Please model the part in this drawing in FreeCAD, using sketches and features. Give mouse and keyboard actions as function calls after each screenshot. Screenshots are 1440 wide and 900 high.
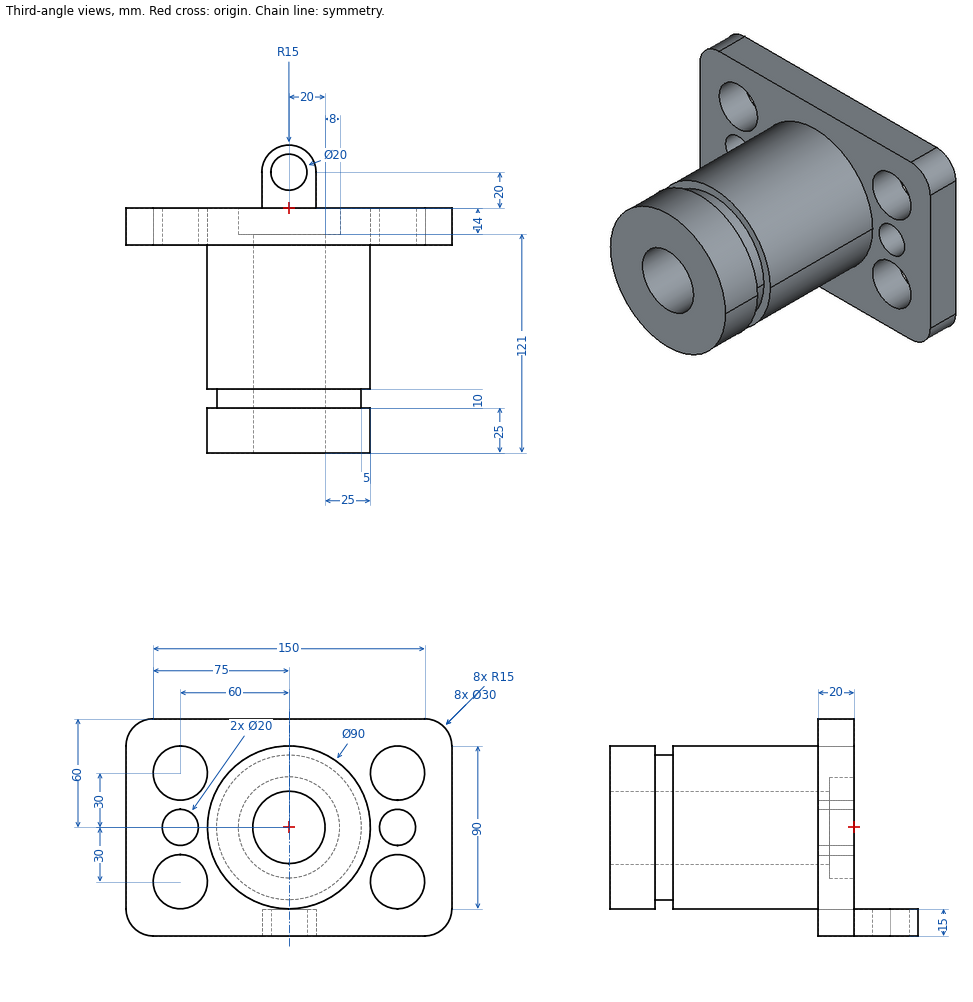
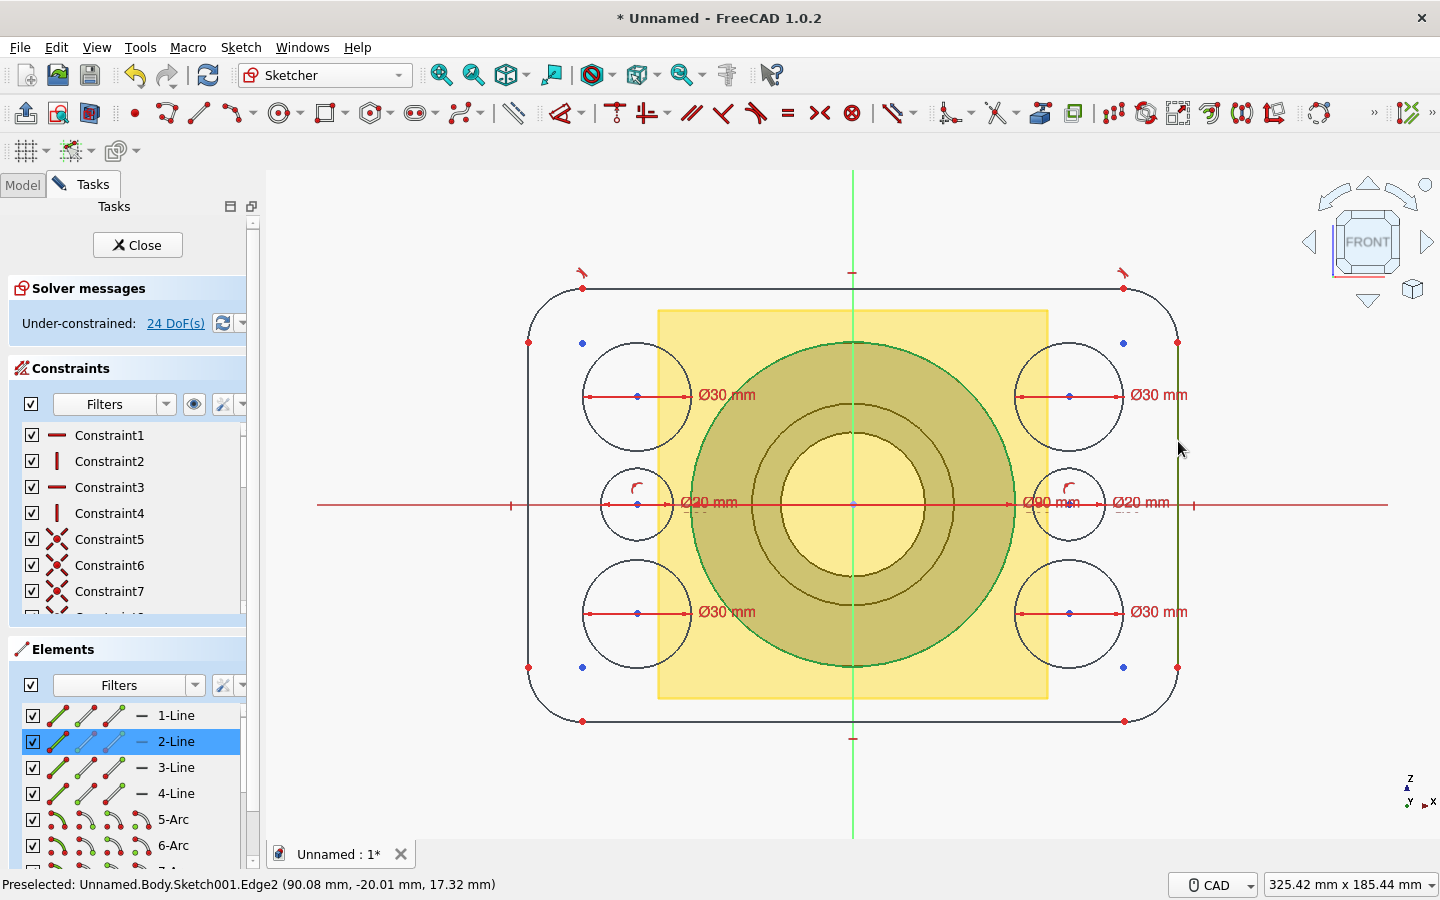
click(1172, 318)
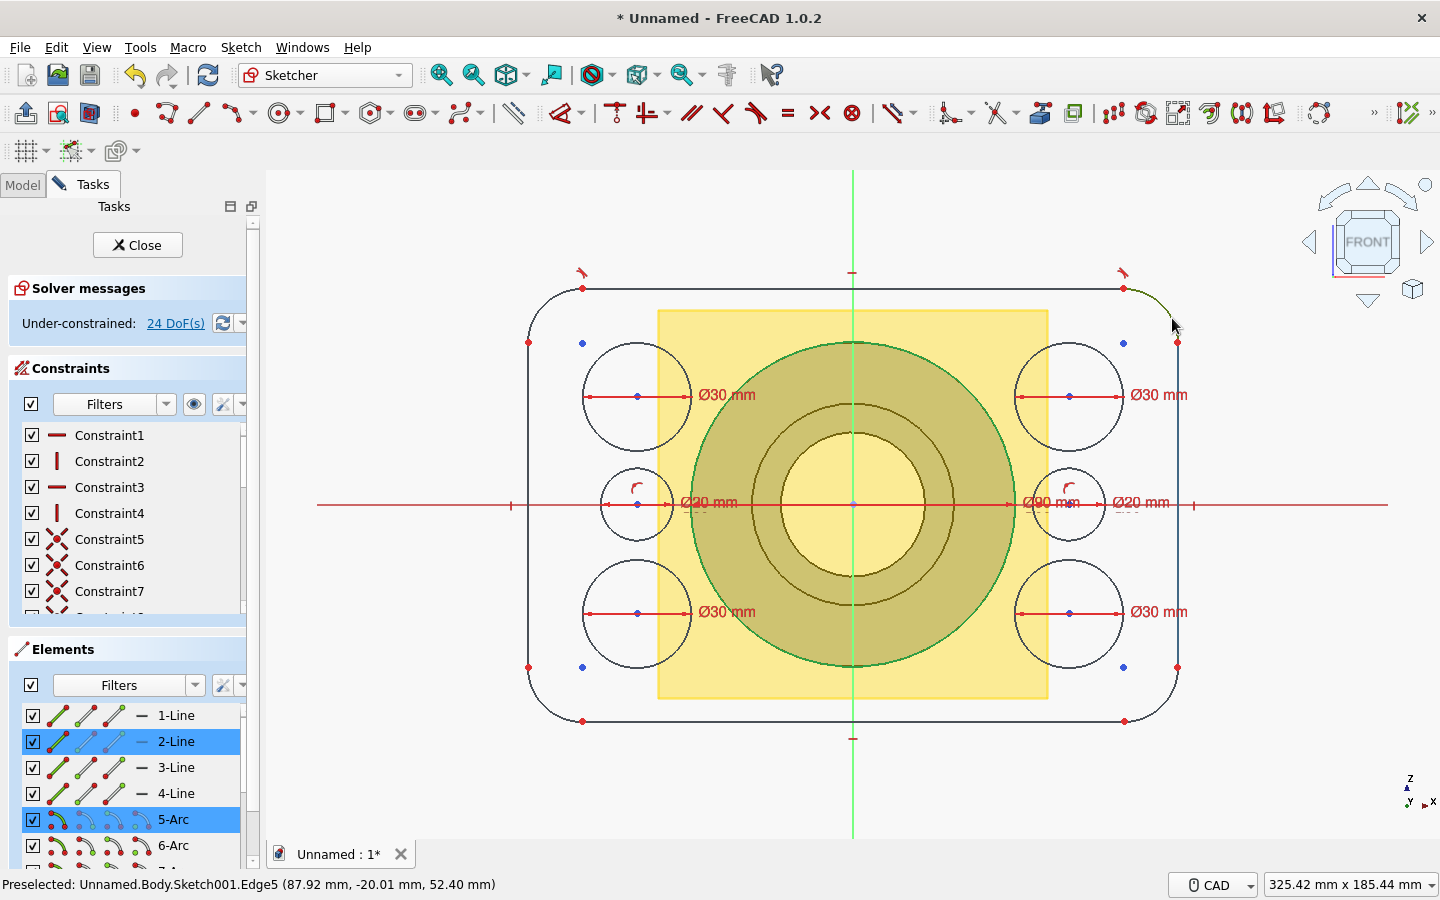
click(756, 114)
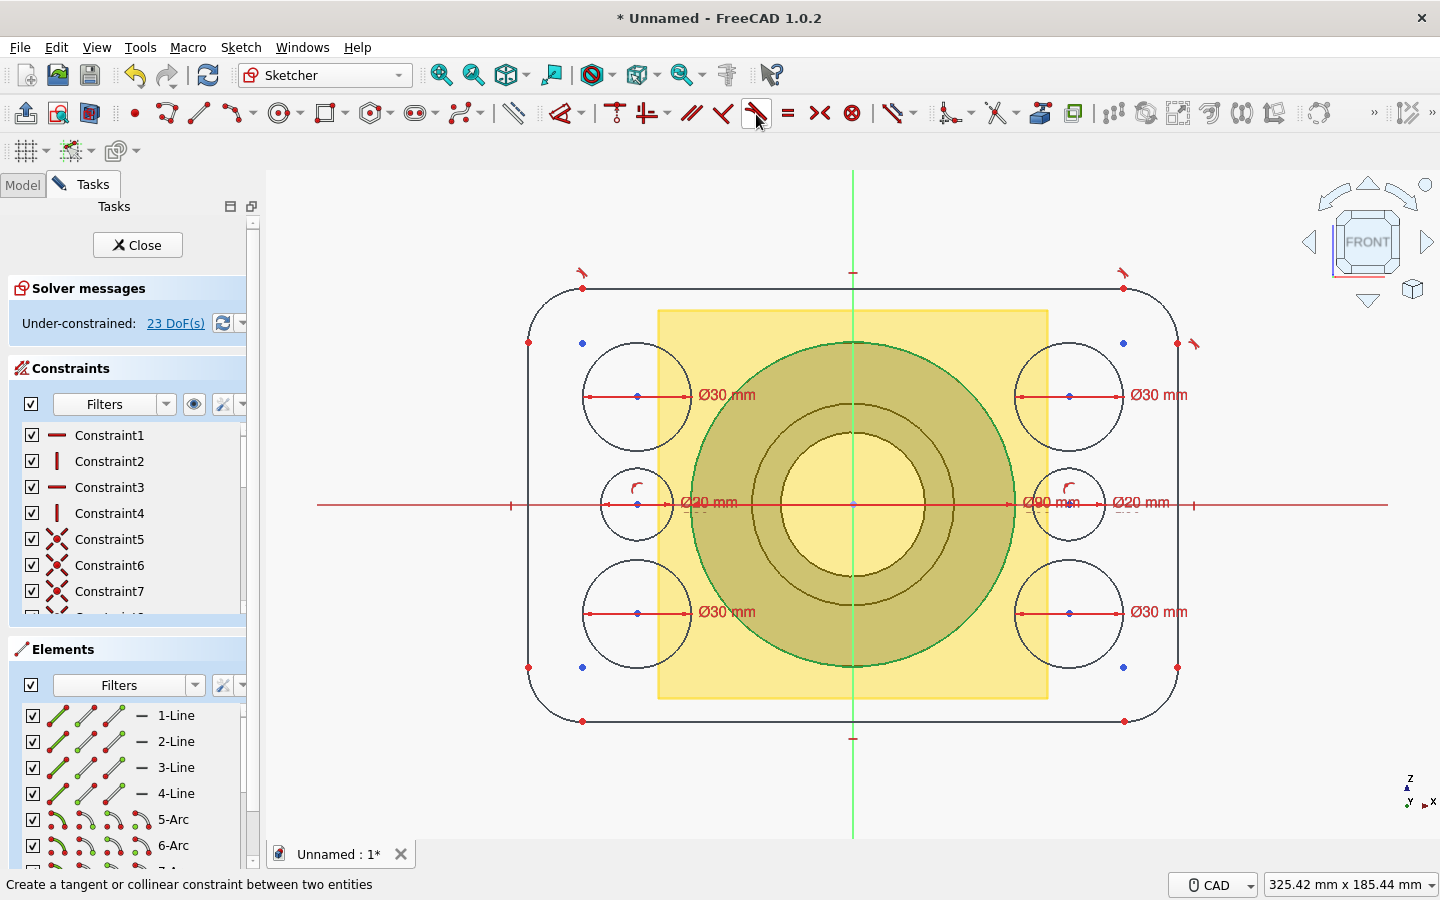
click(1178, 441)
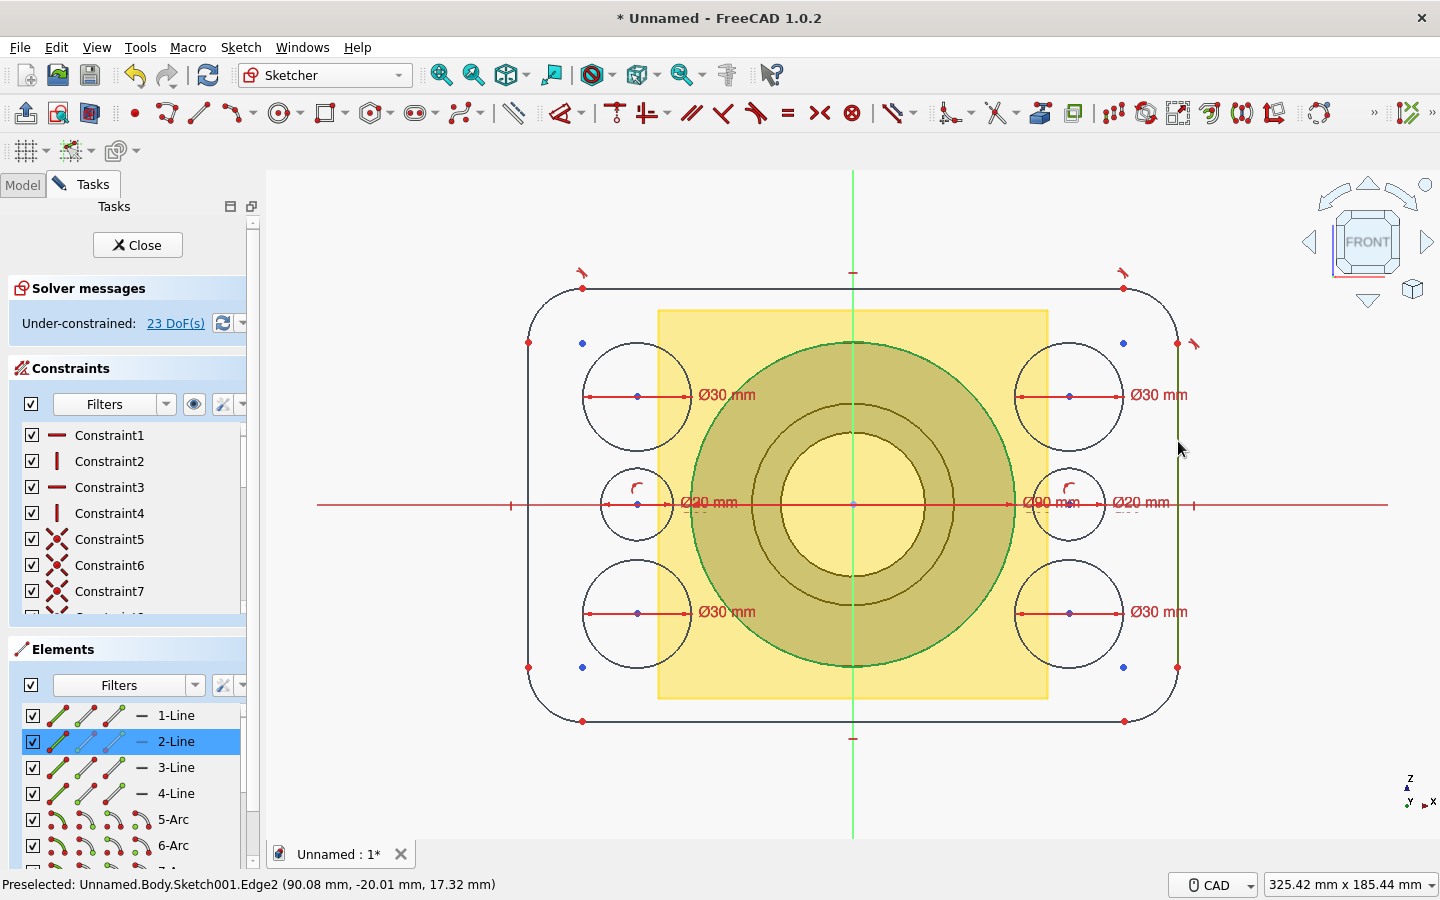
click(1148, 716)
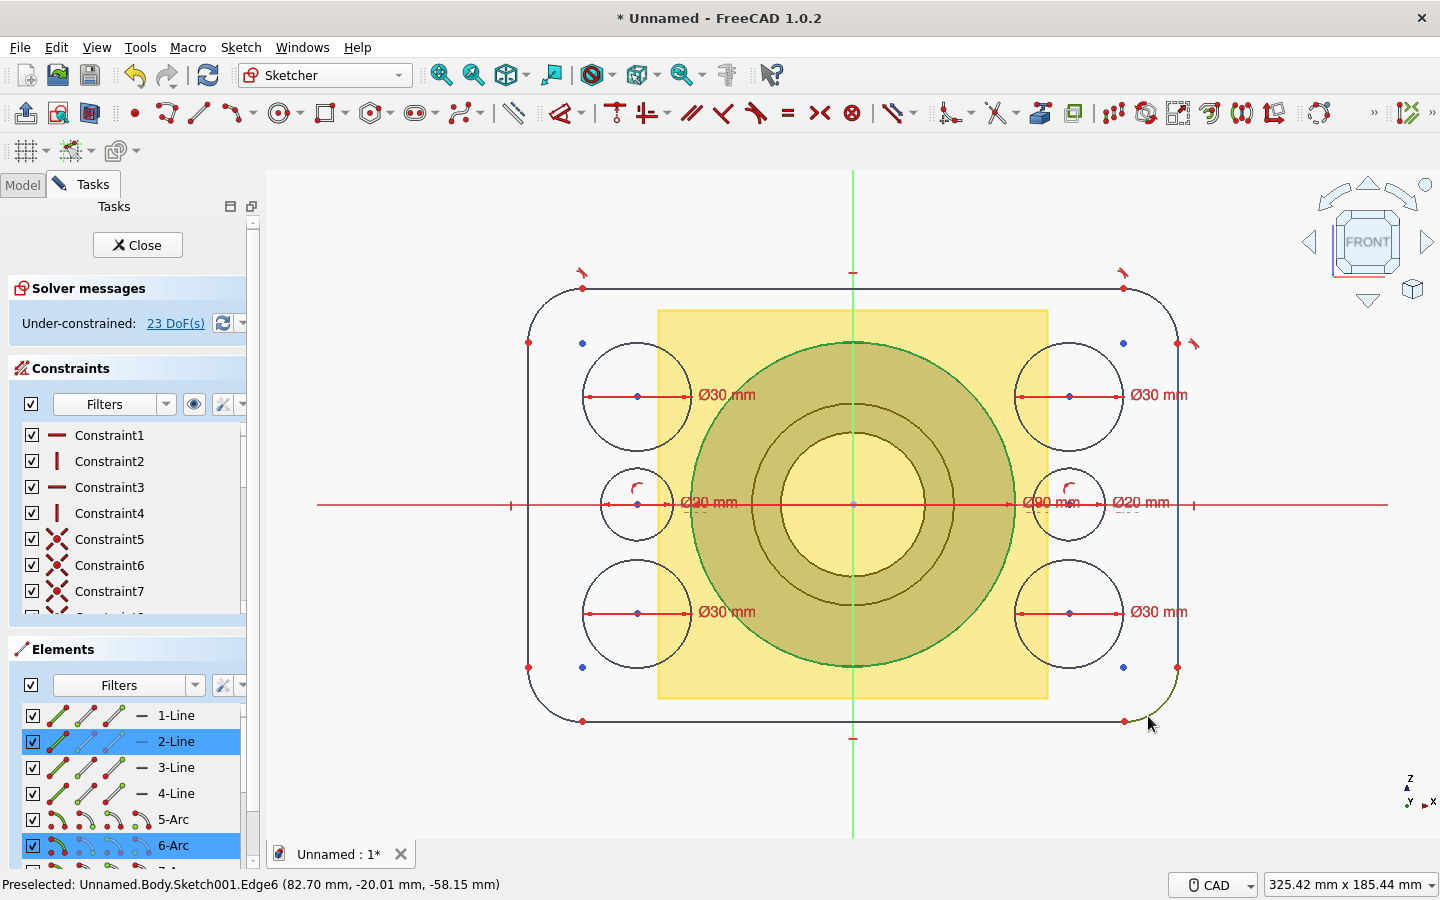
click(756, 114)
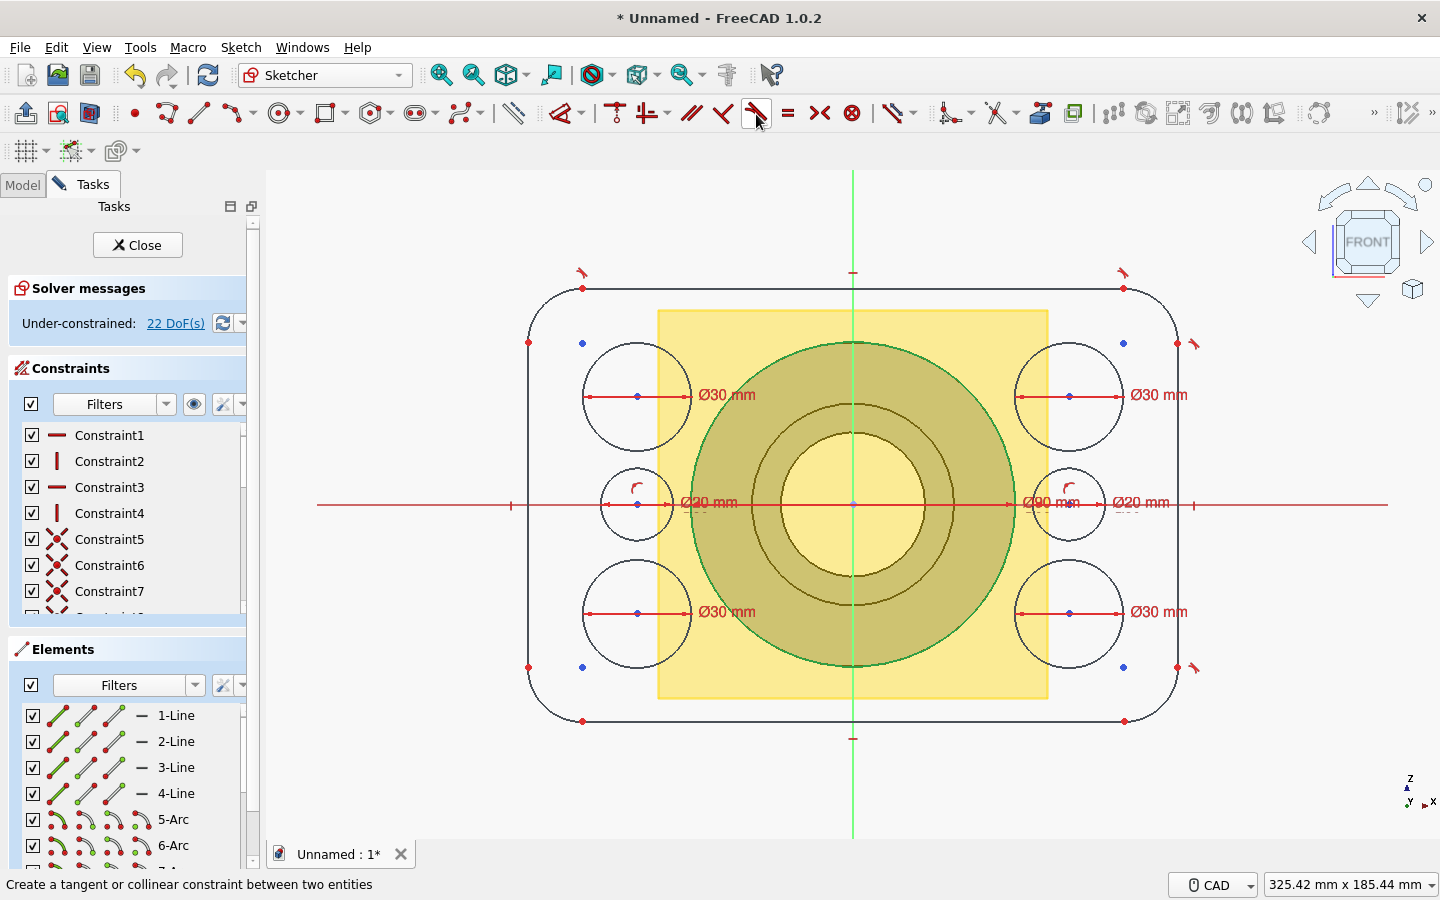
click(961, 722)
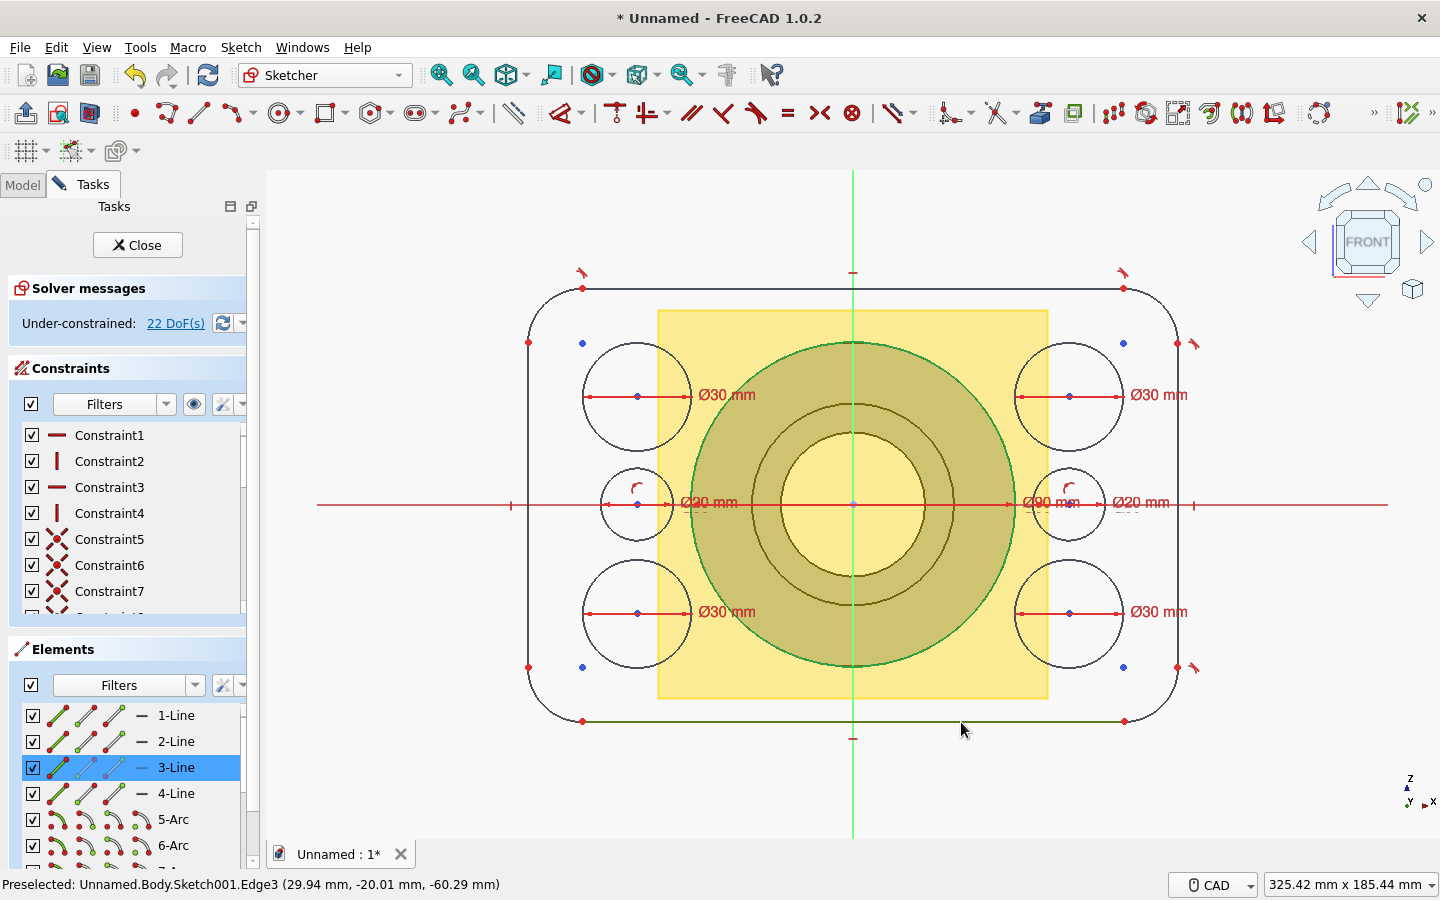
click(1149, 716)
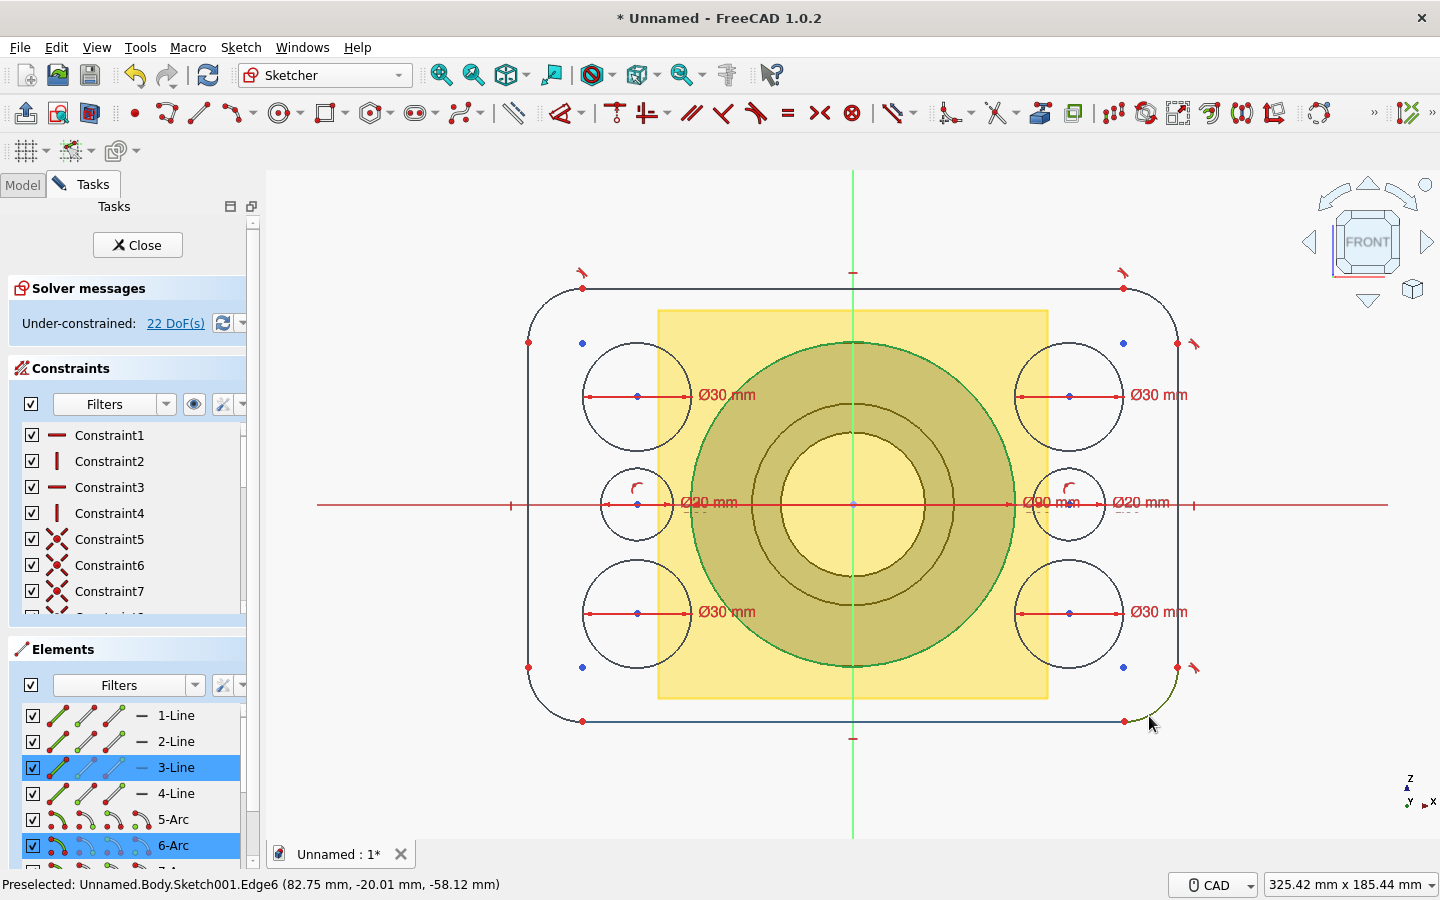
key(t)